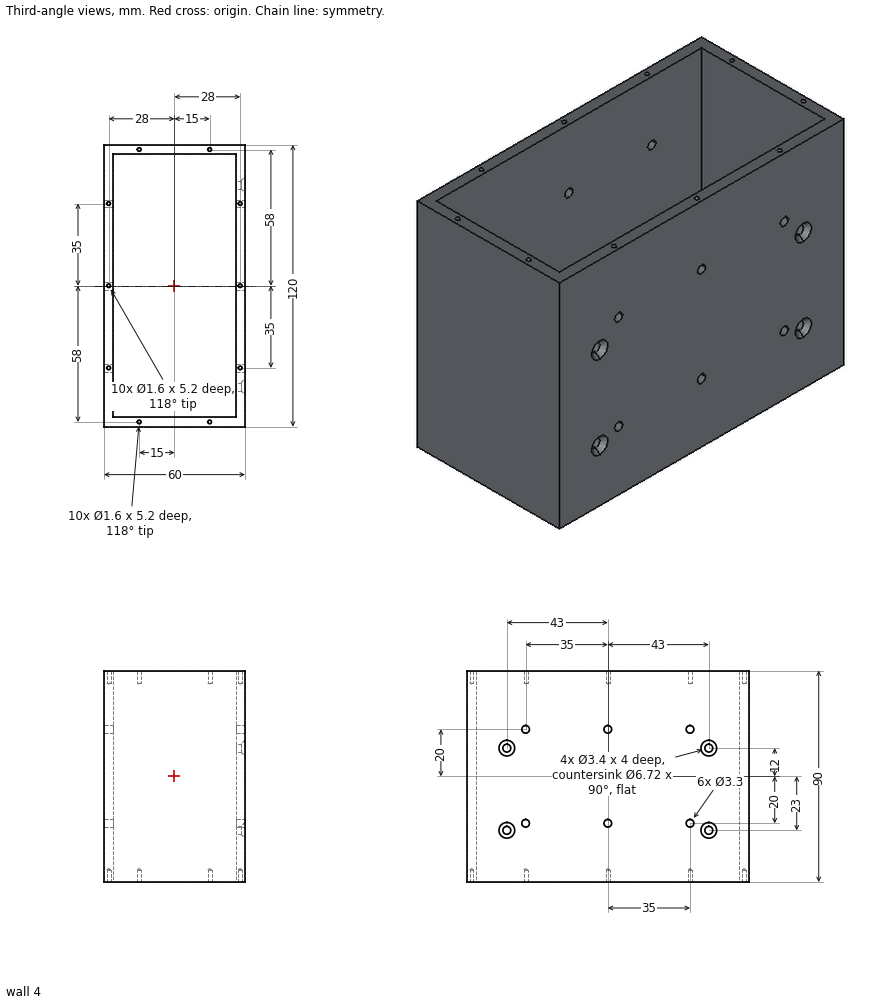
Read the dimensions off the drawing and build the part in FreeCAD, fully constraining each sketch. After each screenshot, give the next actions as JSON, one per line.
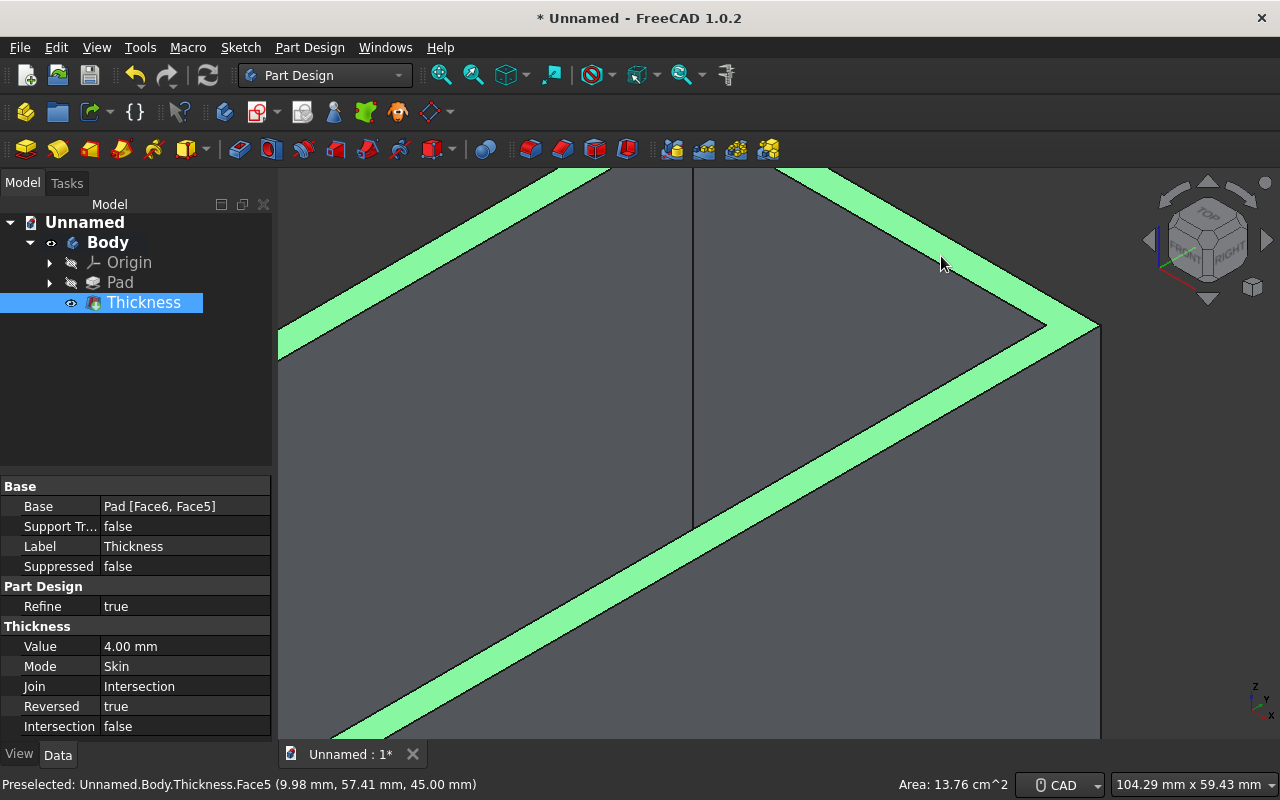
{"action": "left_click", "coordinate": [258, 112]}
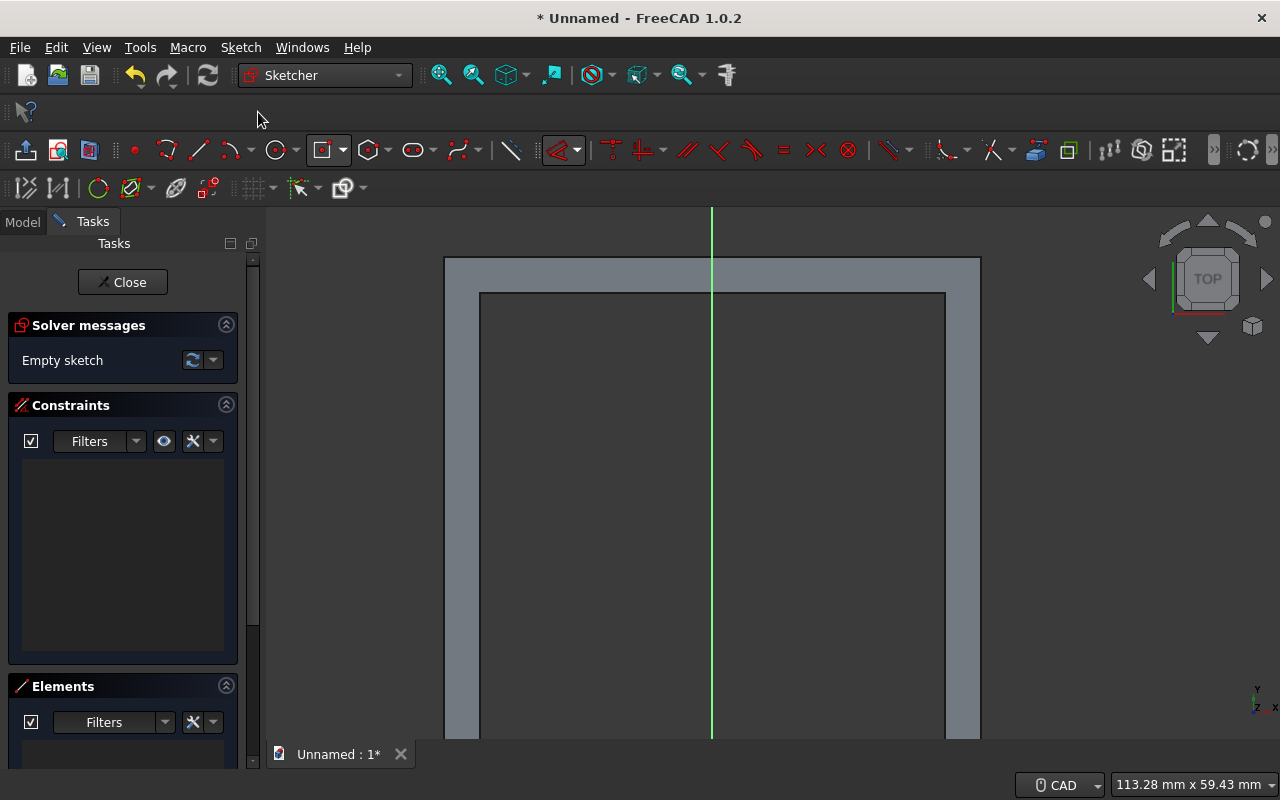
{"action": "scroll", "coordinate": [701, 335], "scroll_direction": "down", "scroll_amount": 6}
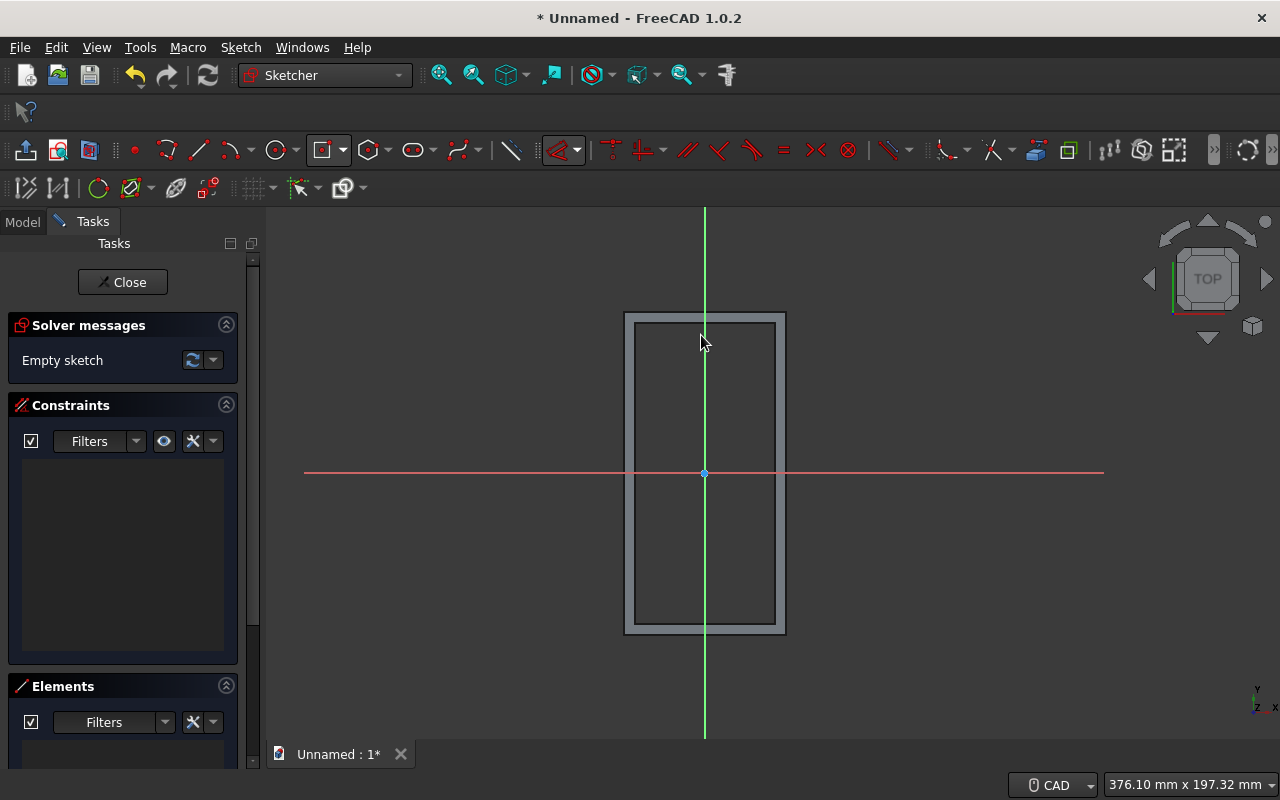
{"action": "left_click", "coordinate": [276, 150]}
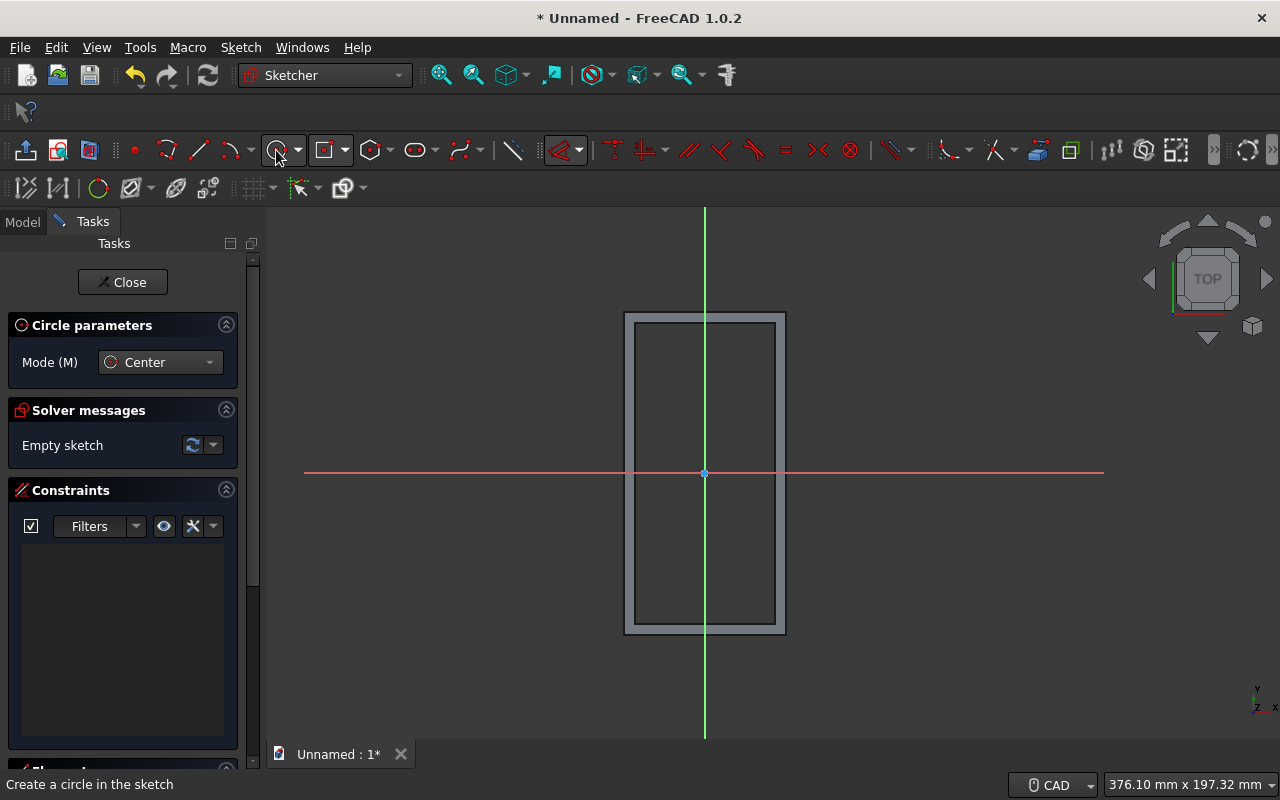
{"action": "scroll", "coordinate": [664, 630], "scroll_direction": "up", "scroll_amount": 12}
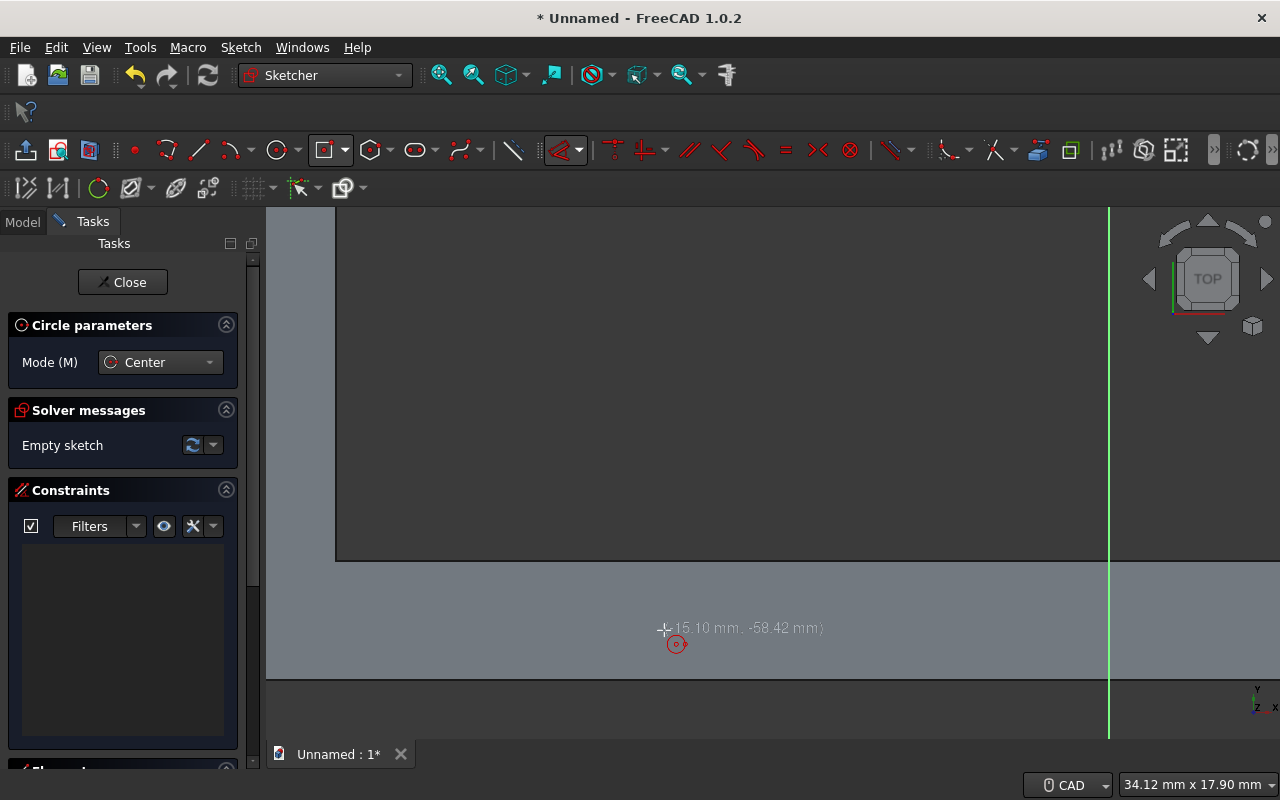
{"action": "scroll", "coordinate": [664, 630], "scroll_direction": "down", "scroll_amount": 12}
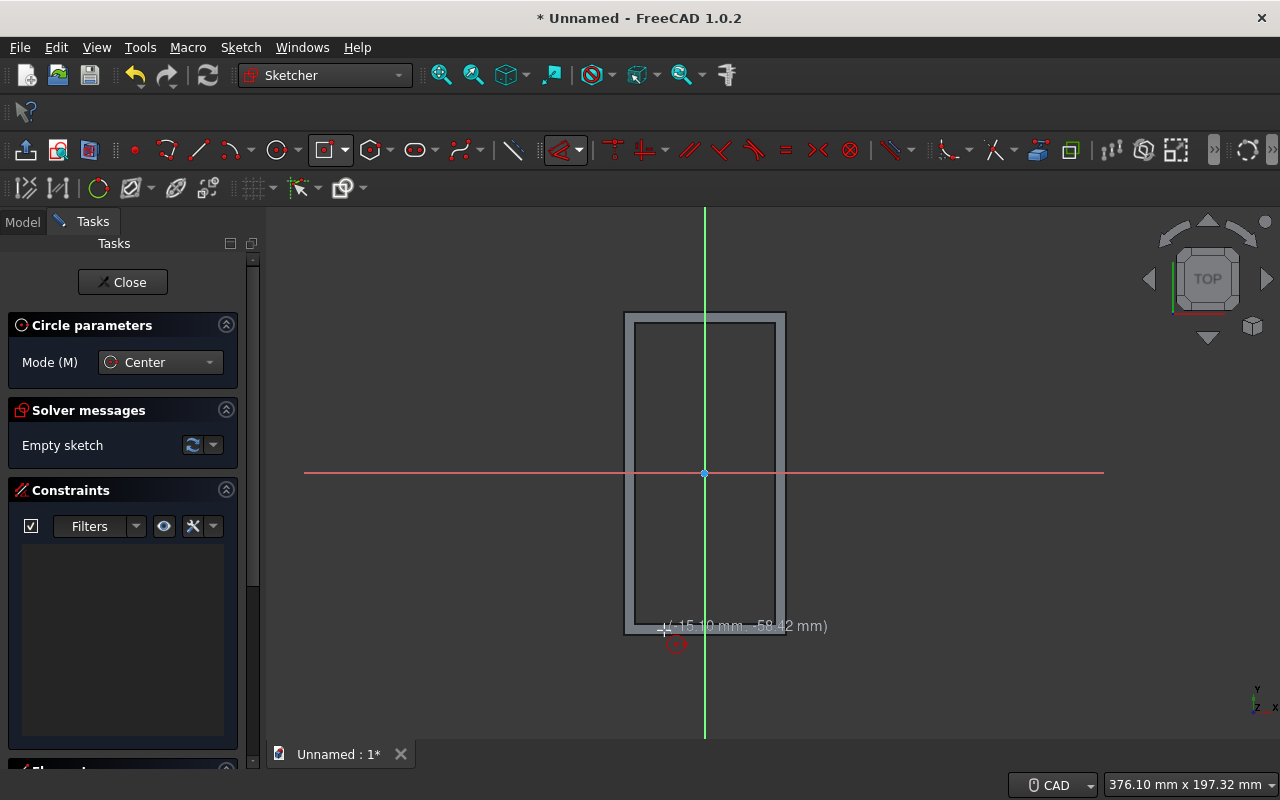
{"action": "left_click", "coordinate": [664, 630]}
{"action": "mouse_move", "coordinate": [666, 628]}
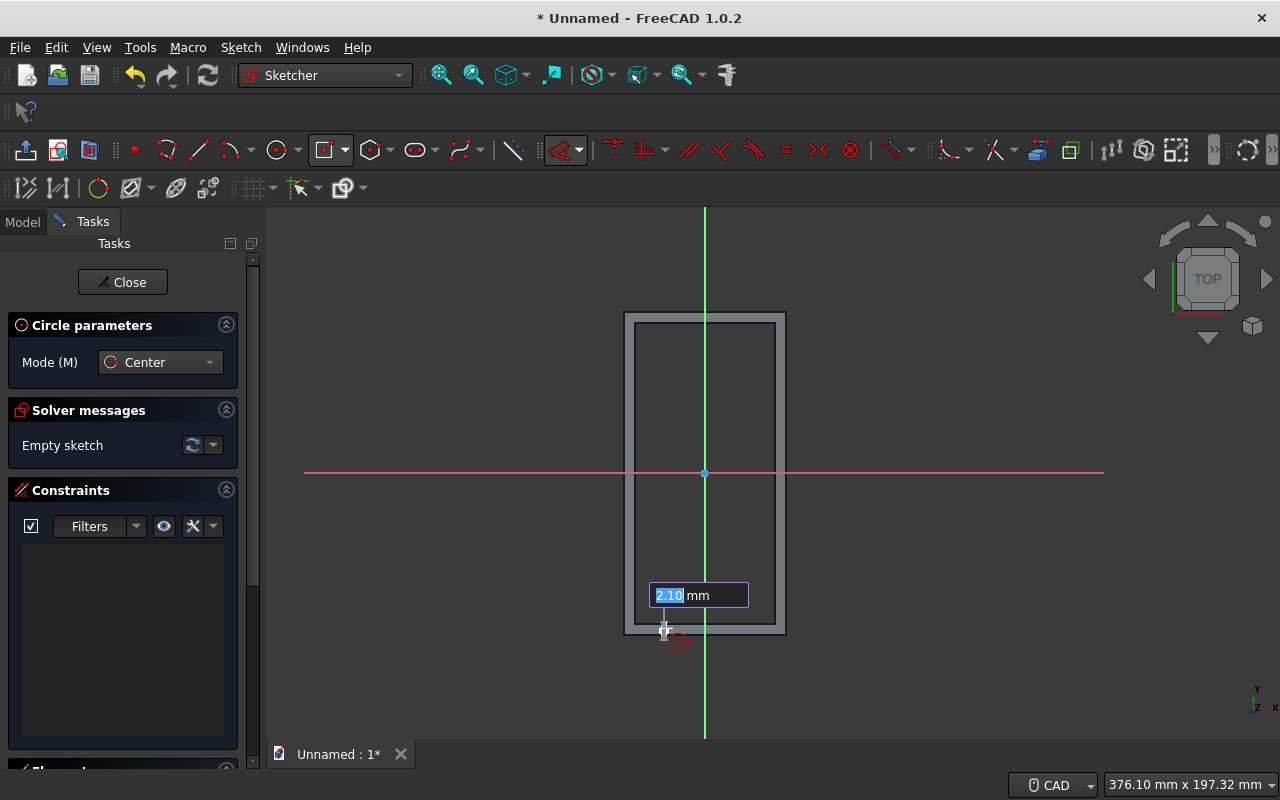
{"action": "type", "text": "1.6"}
{"action": "key", "text": "Return"}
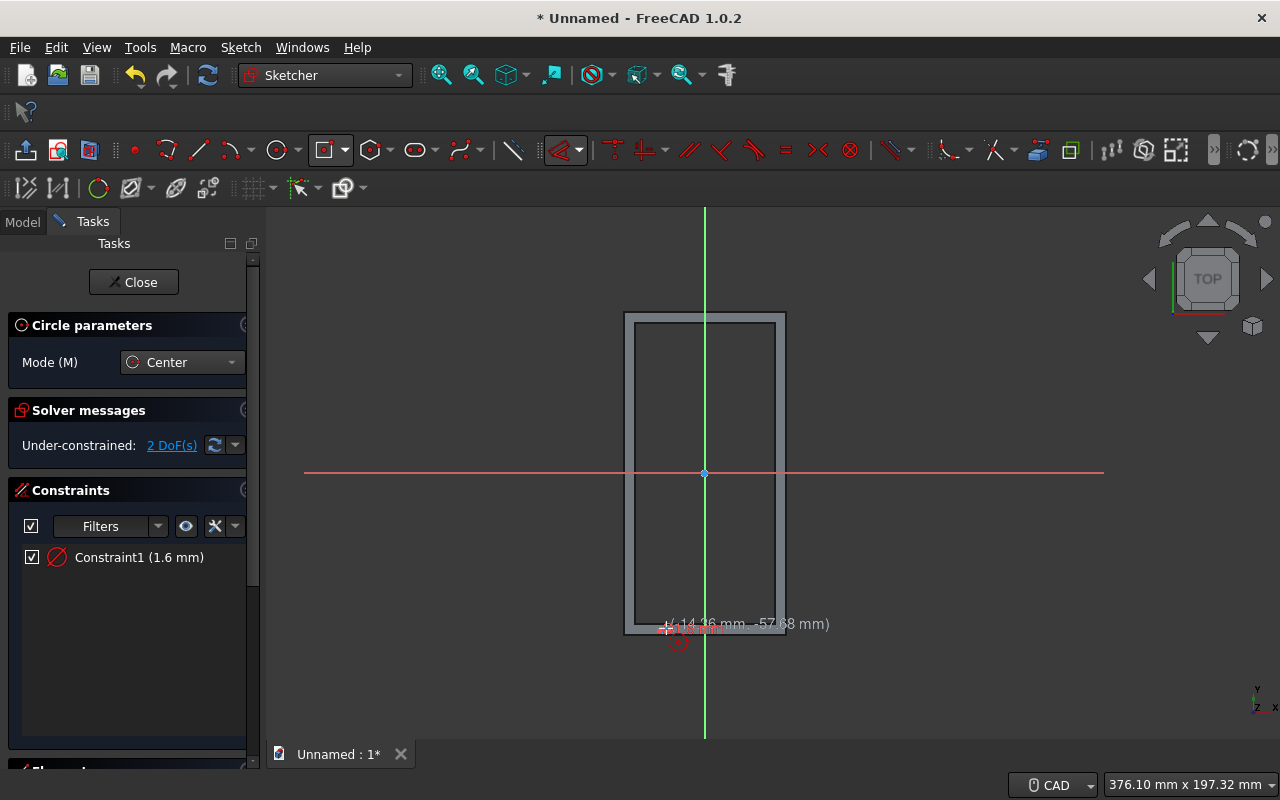
{"action": "scroll", "coordinate": [629, 473], "scroll_direction": "up", "scroll_amount": 12}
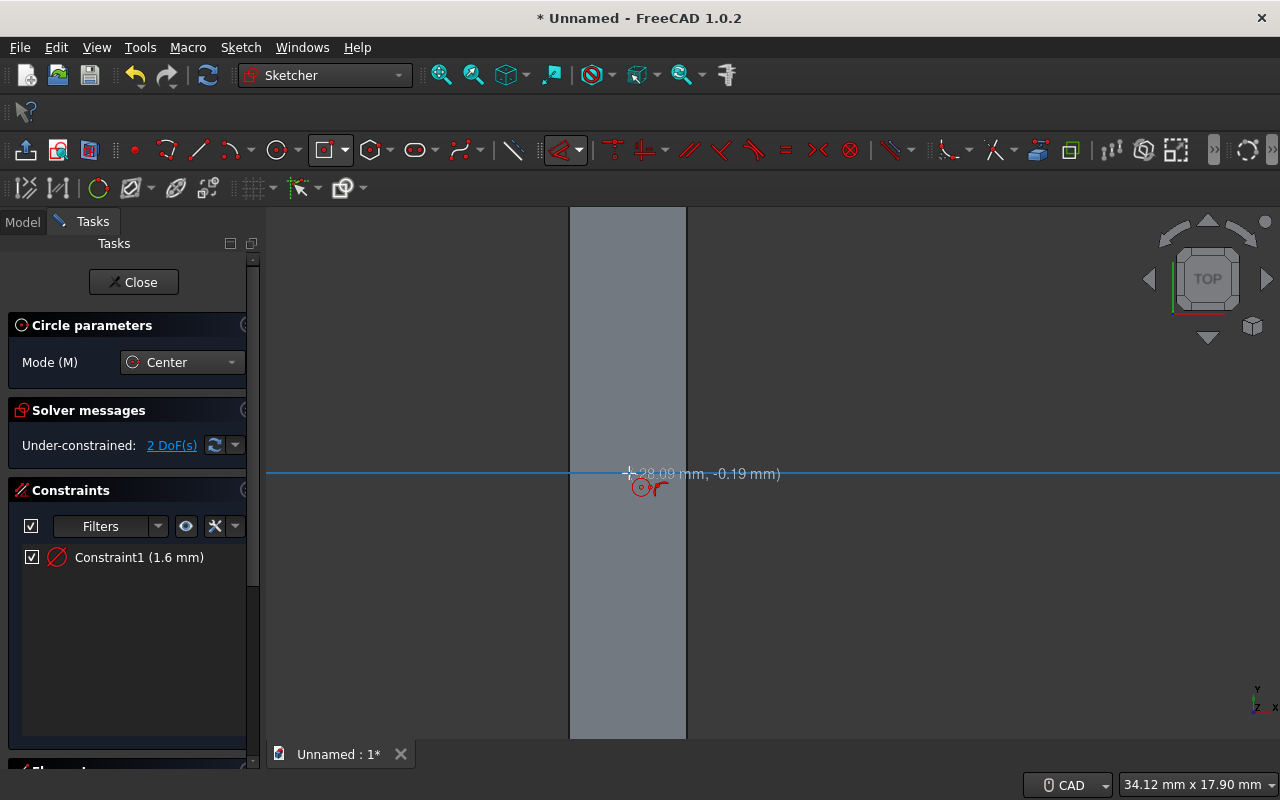
{"action": "scroll", "coordinate": [629, 473], "scroll_direction": "down", "scroll_amount": 12}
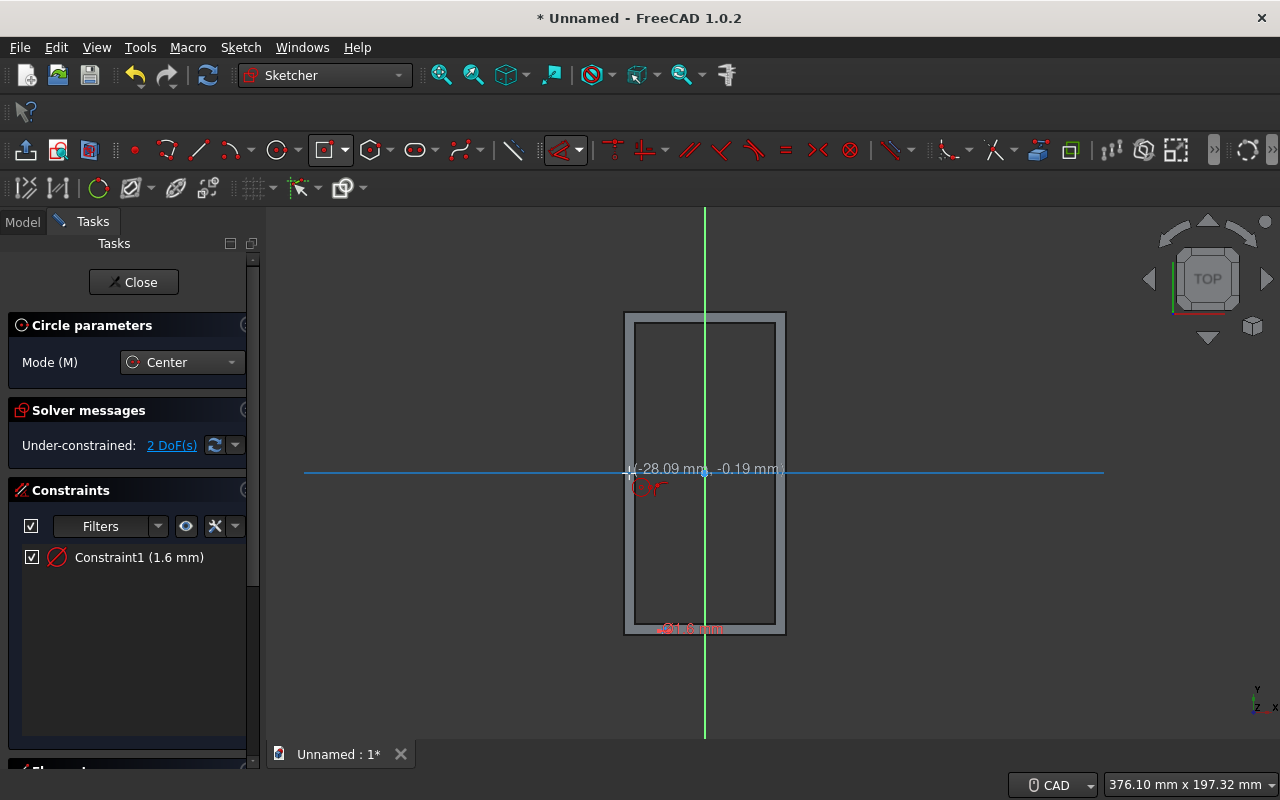
{"action": "left_click", "coordinate": [629, 473]}